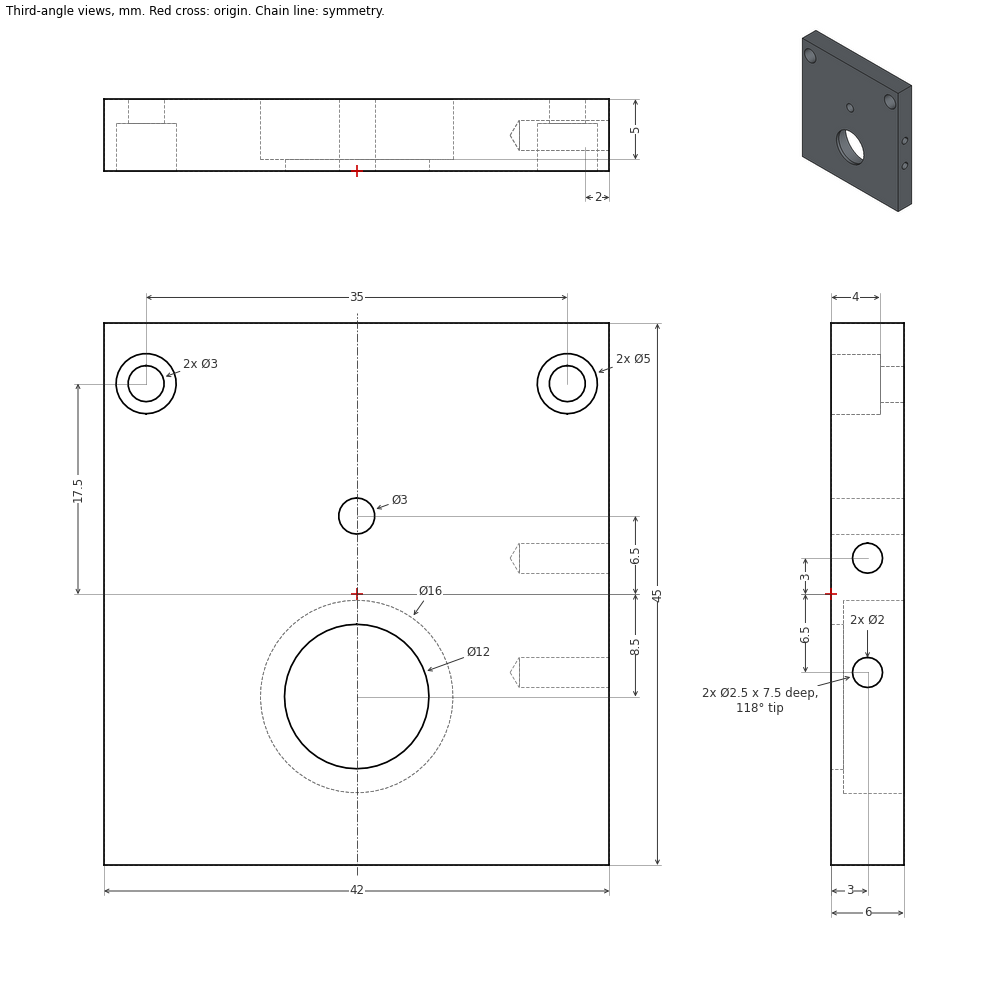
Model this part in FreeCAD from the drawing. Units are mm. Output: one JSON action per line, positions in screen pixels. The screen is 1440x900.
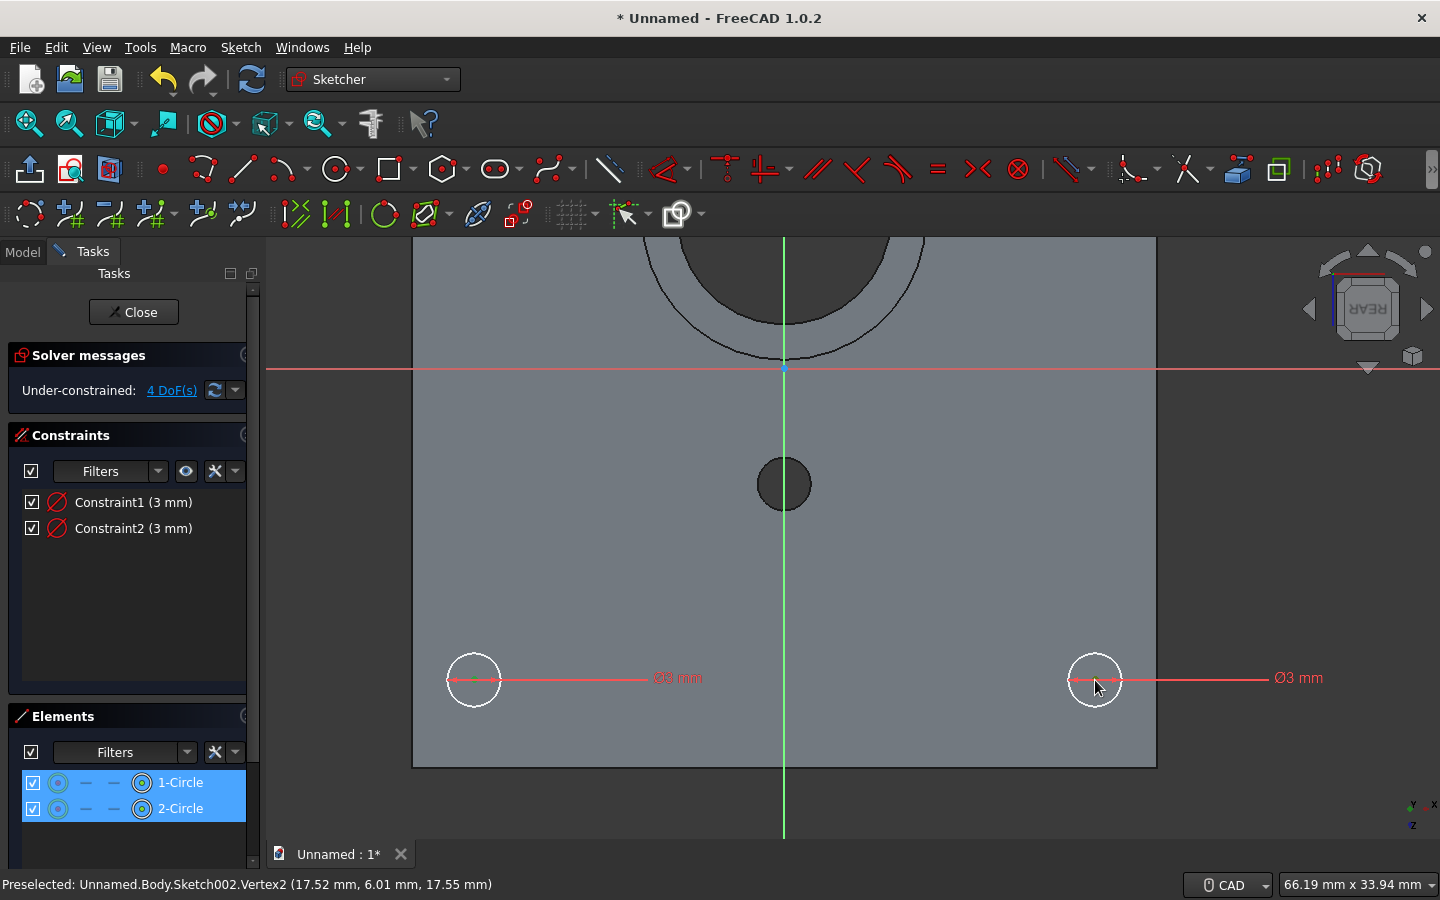
{"action": "left_click", "coordinate": [784, 772]}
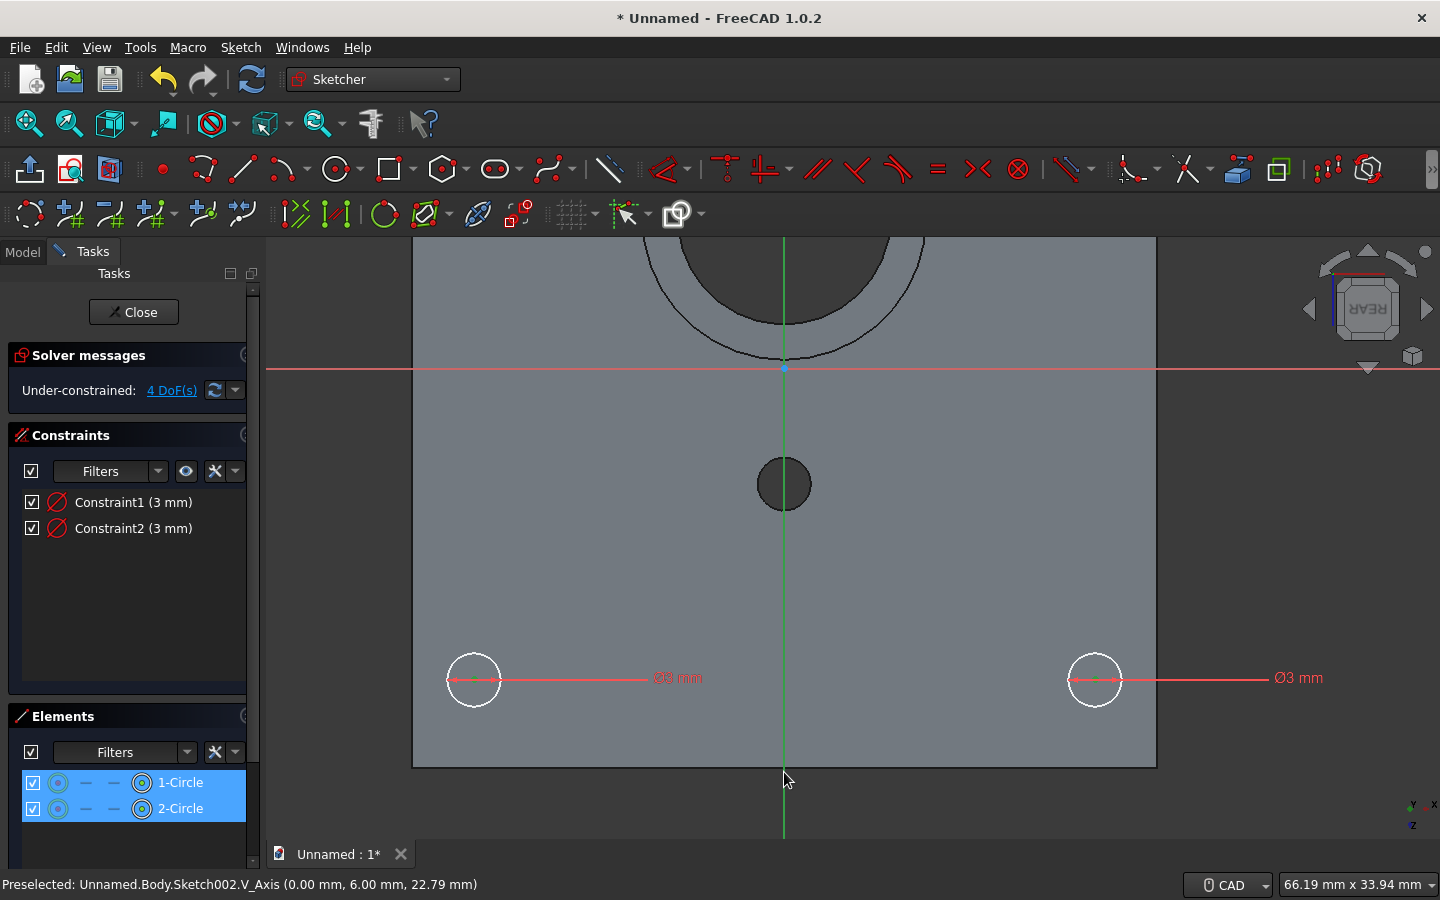
{"action": "key", "text": "s"}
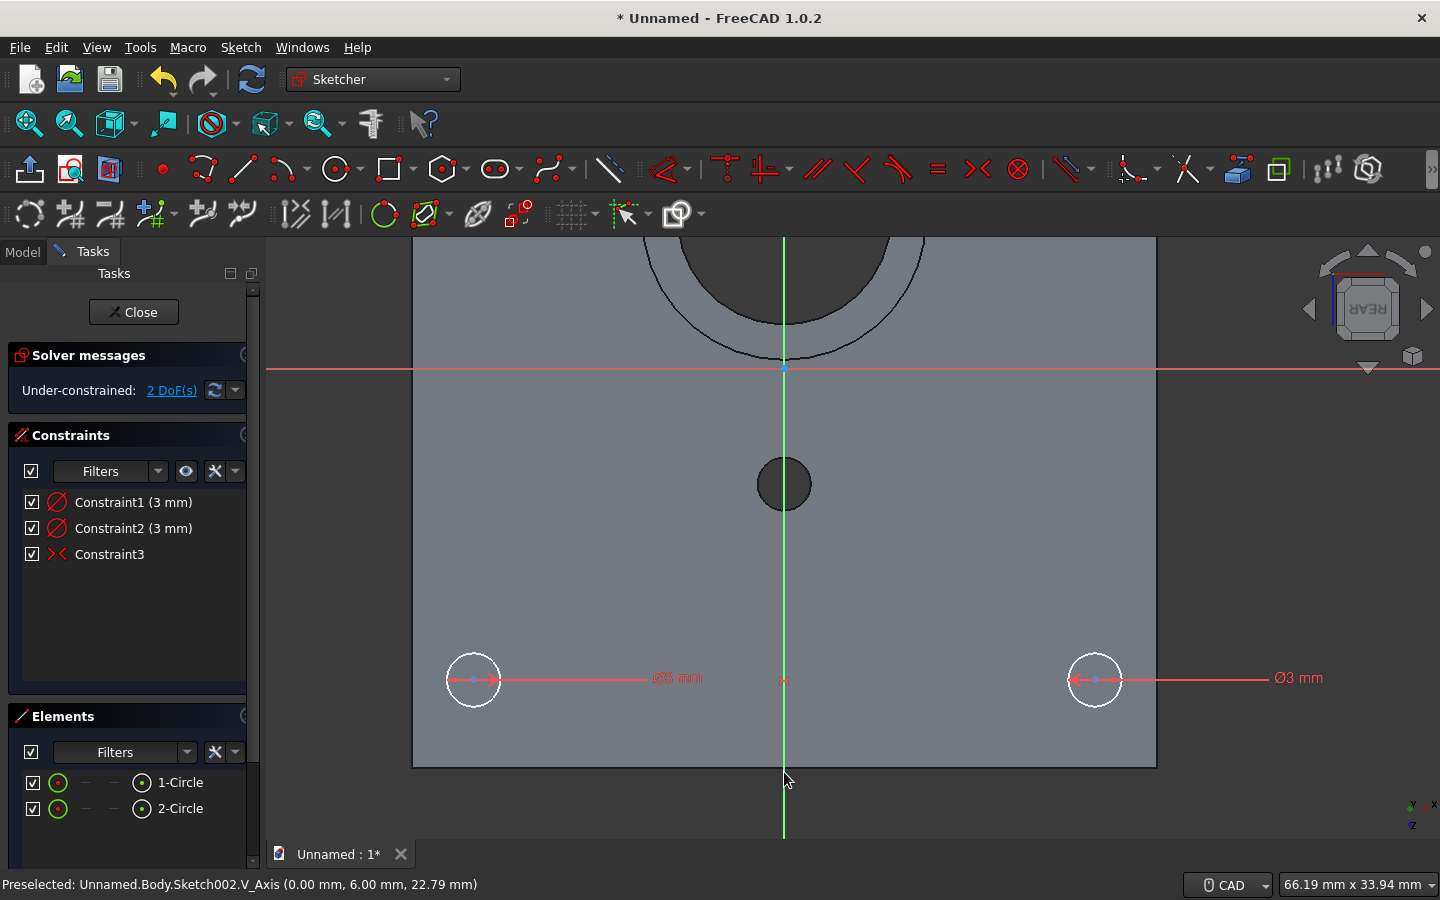
{"action": "left_click", "coordinate": [664, 170]}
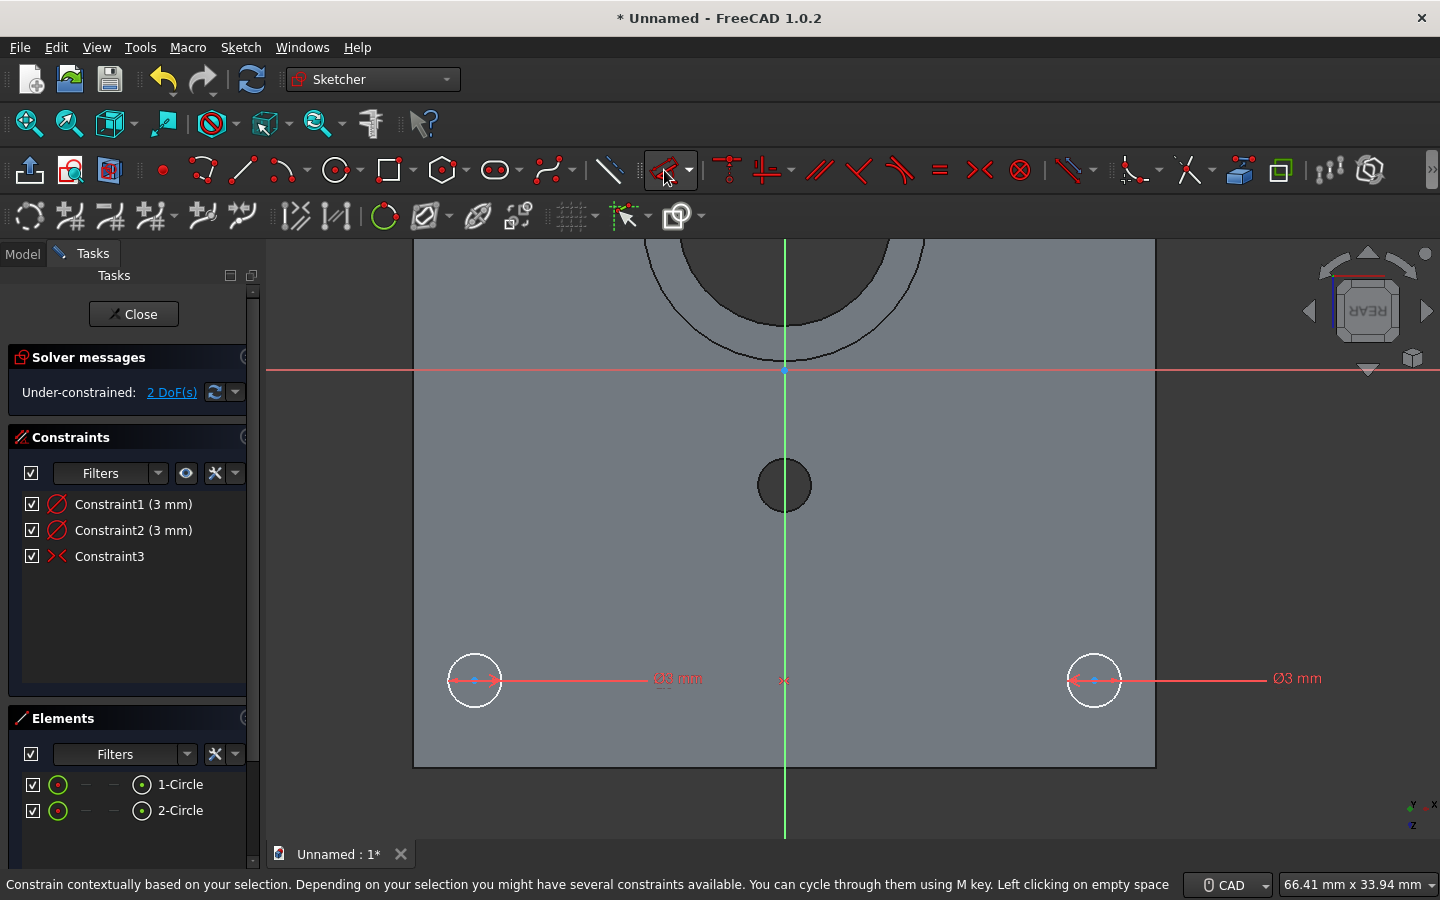
{"action": "left_click", "coordinate": [475, 681]}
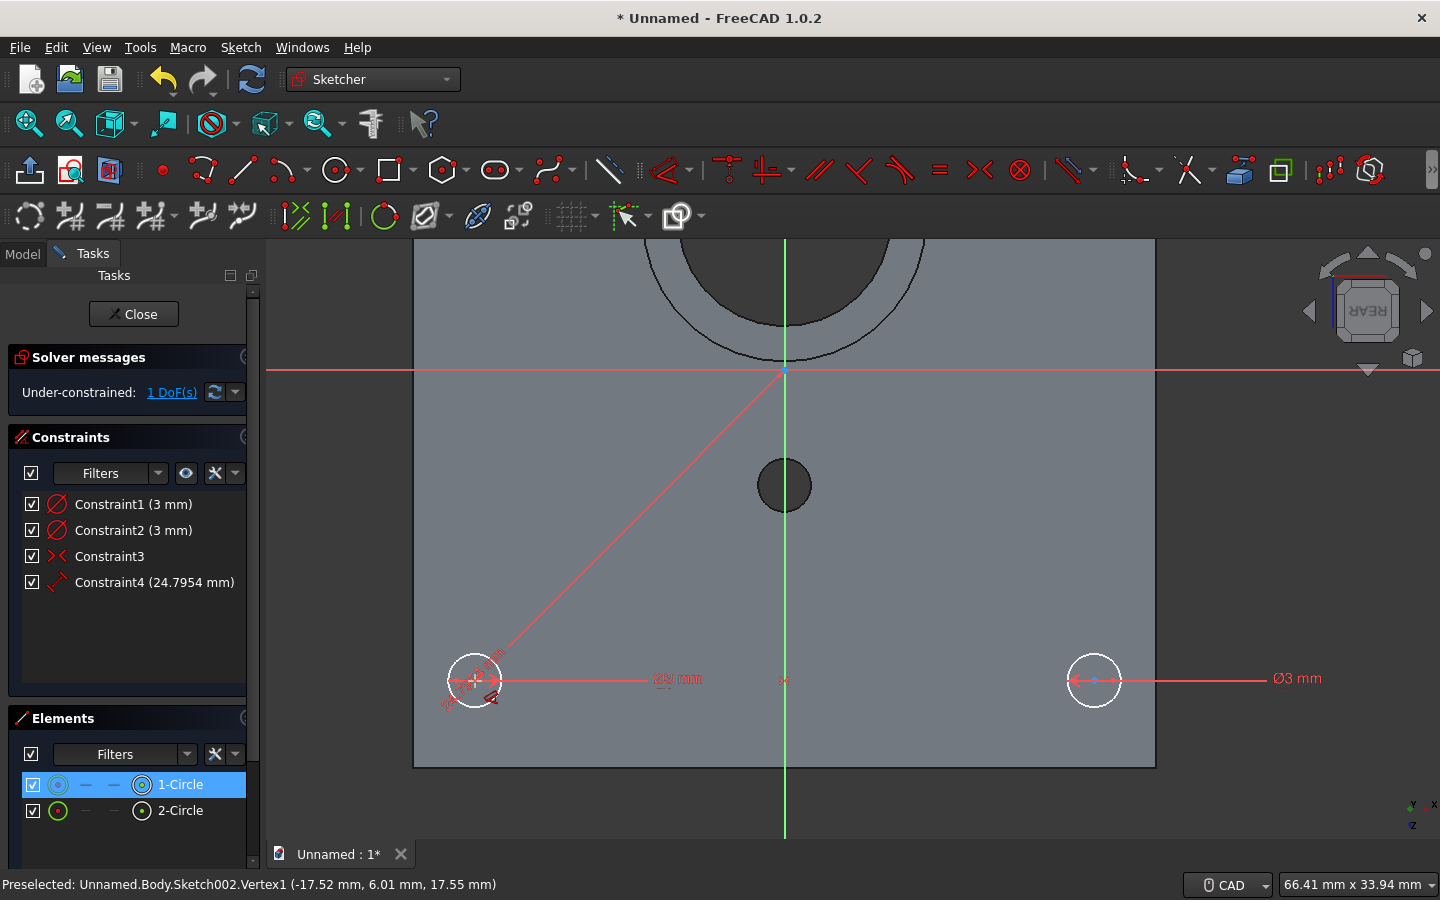
{"action": "left_click", "coordinate": [1094, 681]}
{"action": "left_click", "coordinate": [642, 715]}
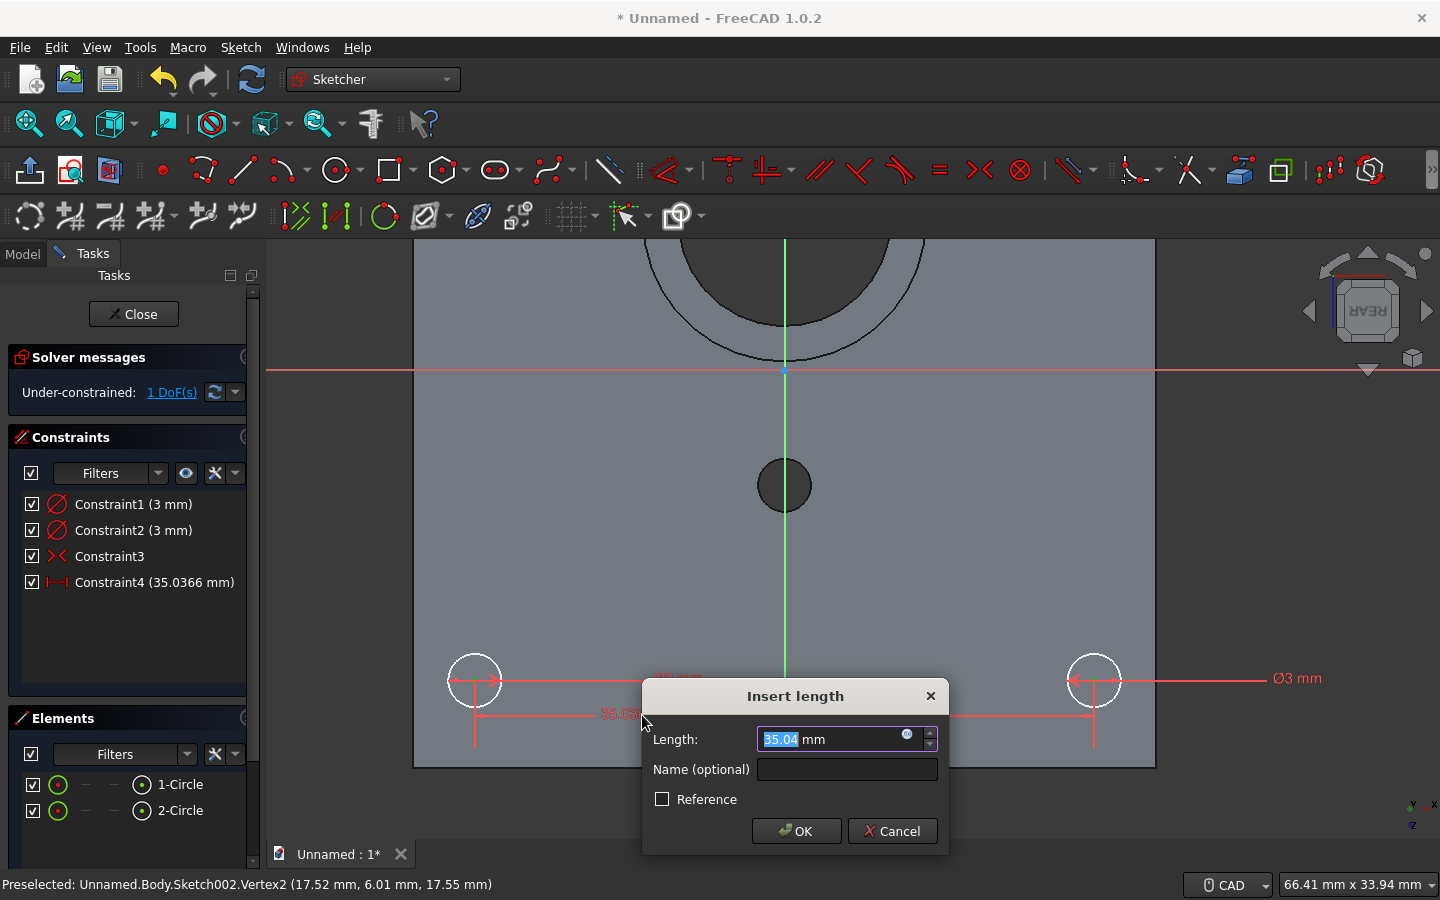
{"action": "type", "text": "35"}
{"action": "key", "text": "Return"}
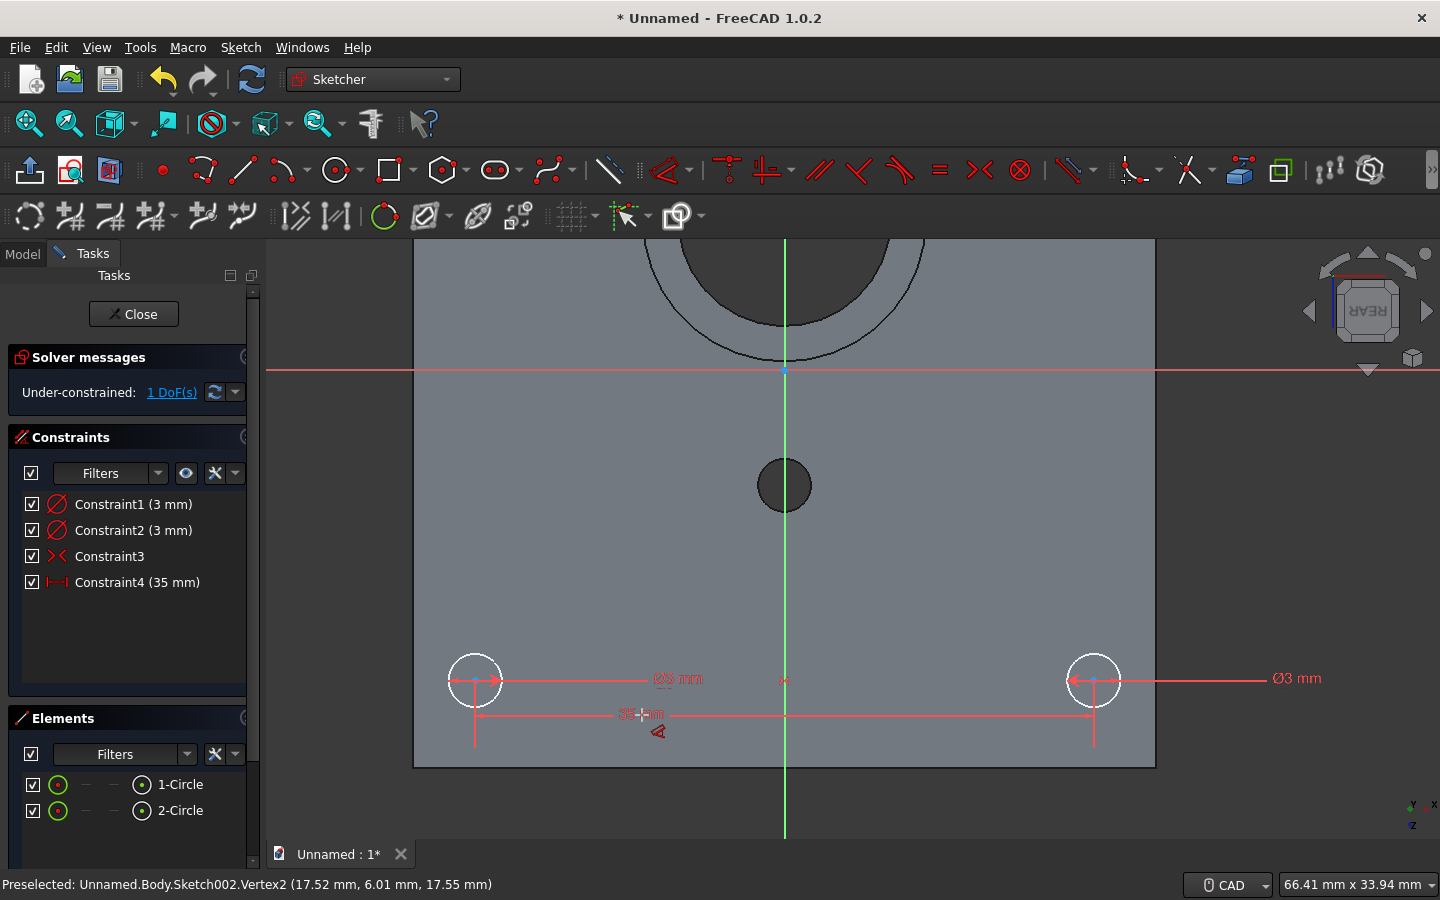
{"action": "left_click", "coordinate": [475, 681]}
{"action": "left_click", "coordinate": [441, 525]}